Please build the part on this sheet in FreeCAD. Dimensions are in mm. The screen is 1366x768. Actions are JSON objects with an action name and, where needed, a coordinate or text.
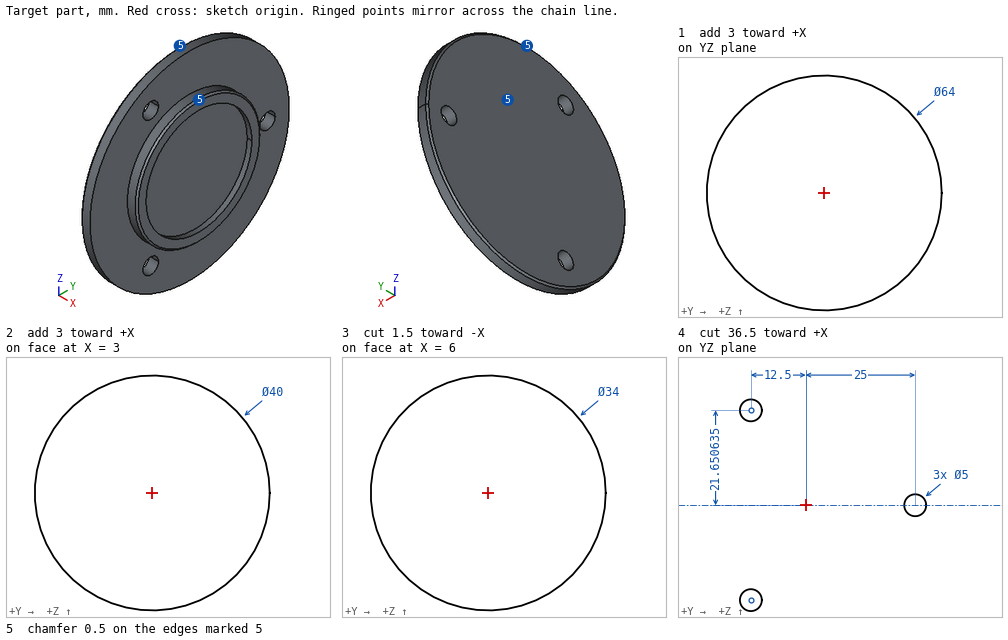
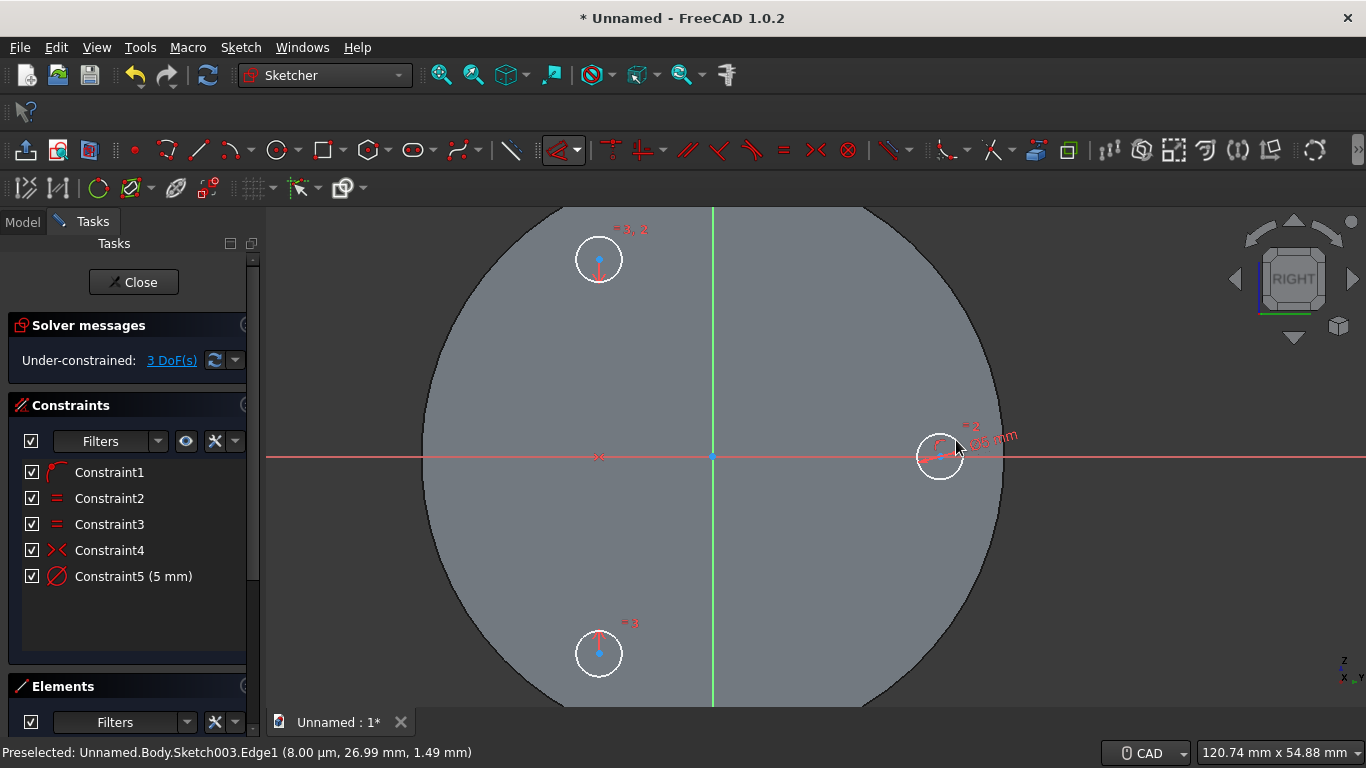
{"action": "left_click", "coordinate": [940, 457]}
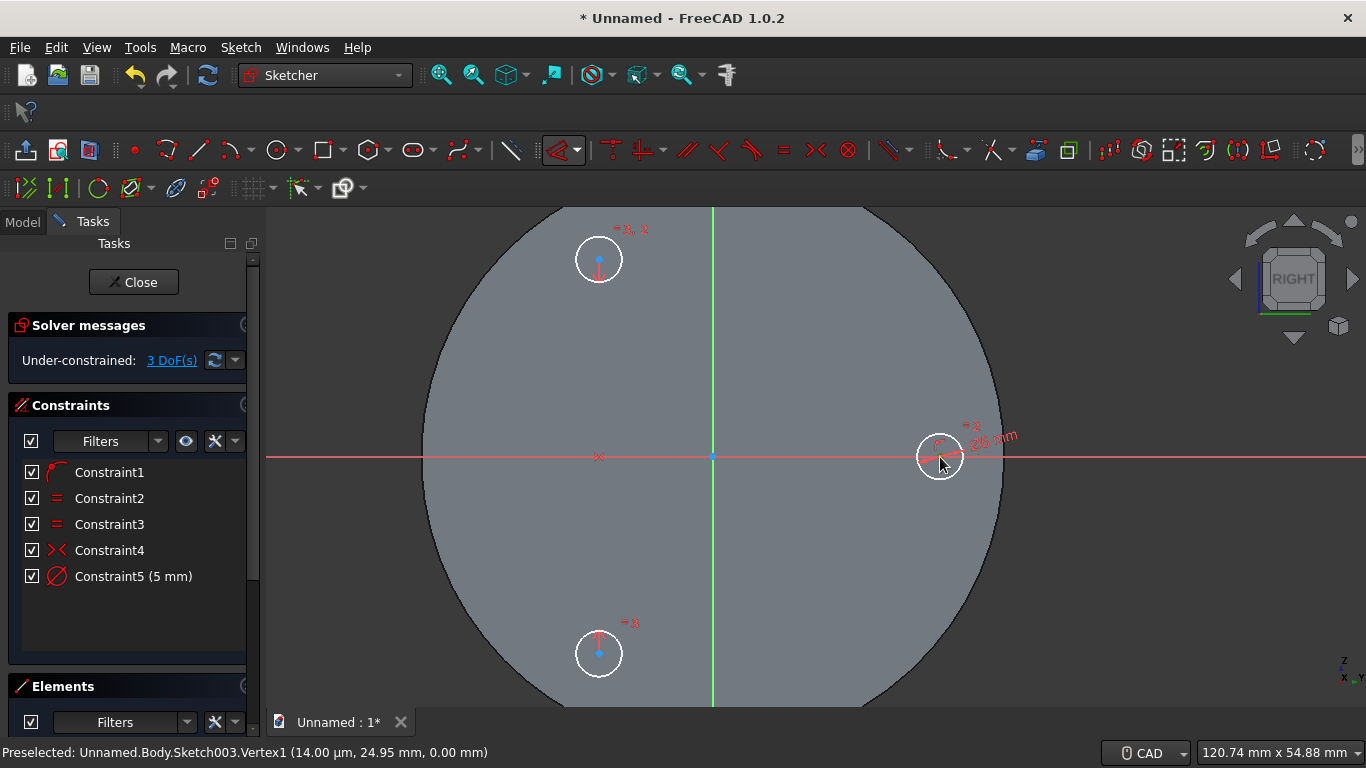
{"action": "key", "text": "l"}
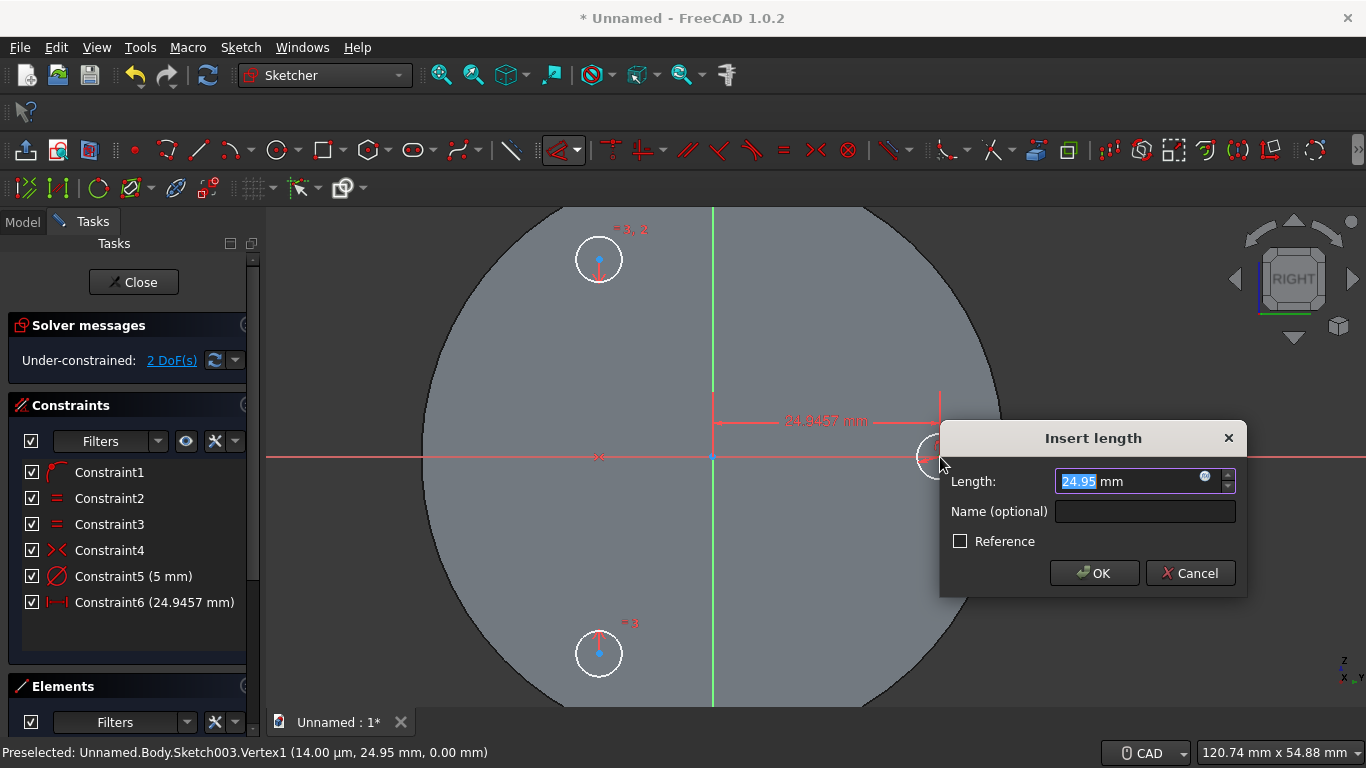
{"action": "type", "text": "25"}
{"action": "key", "text": "Return"}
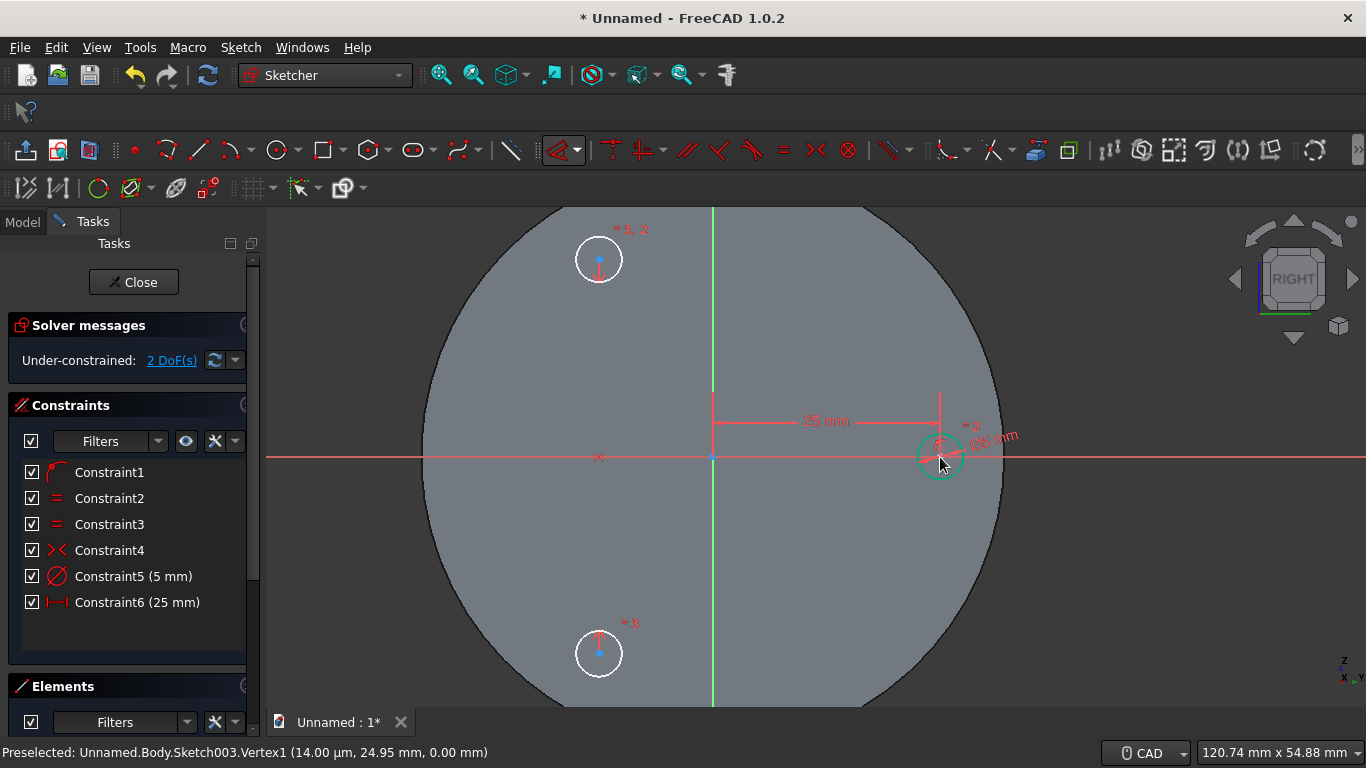
{"action": "left_click", "coordinate": [599, 259]}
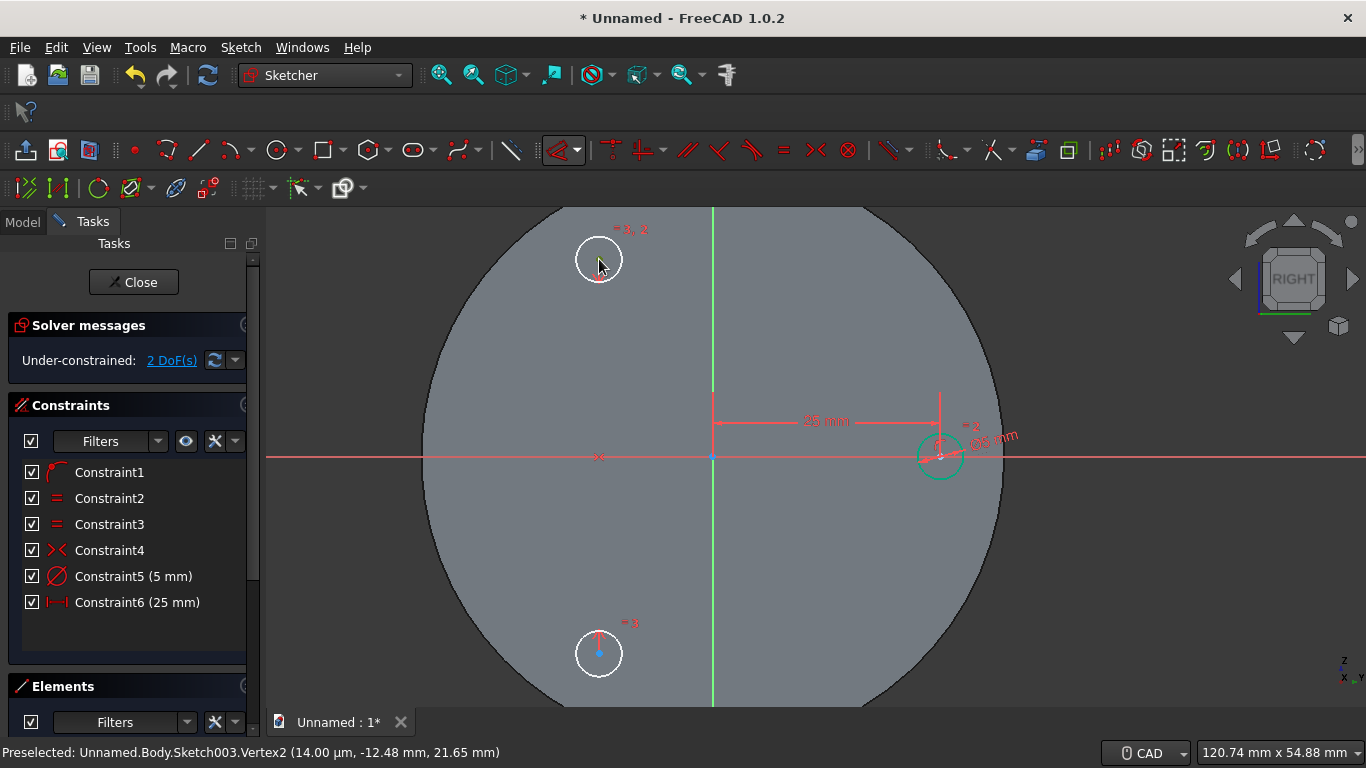
{"action": "left_click", "coordinate": [580, 150]}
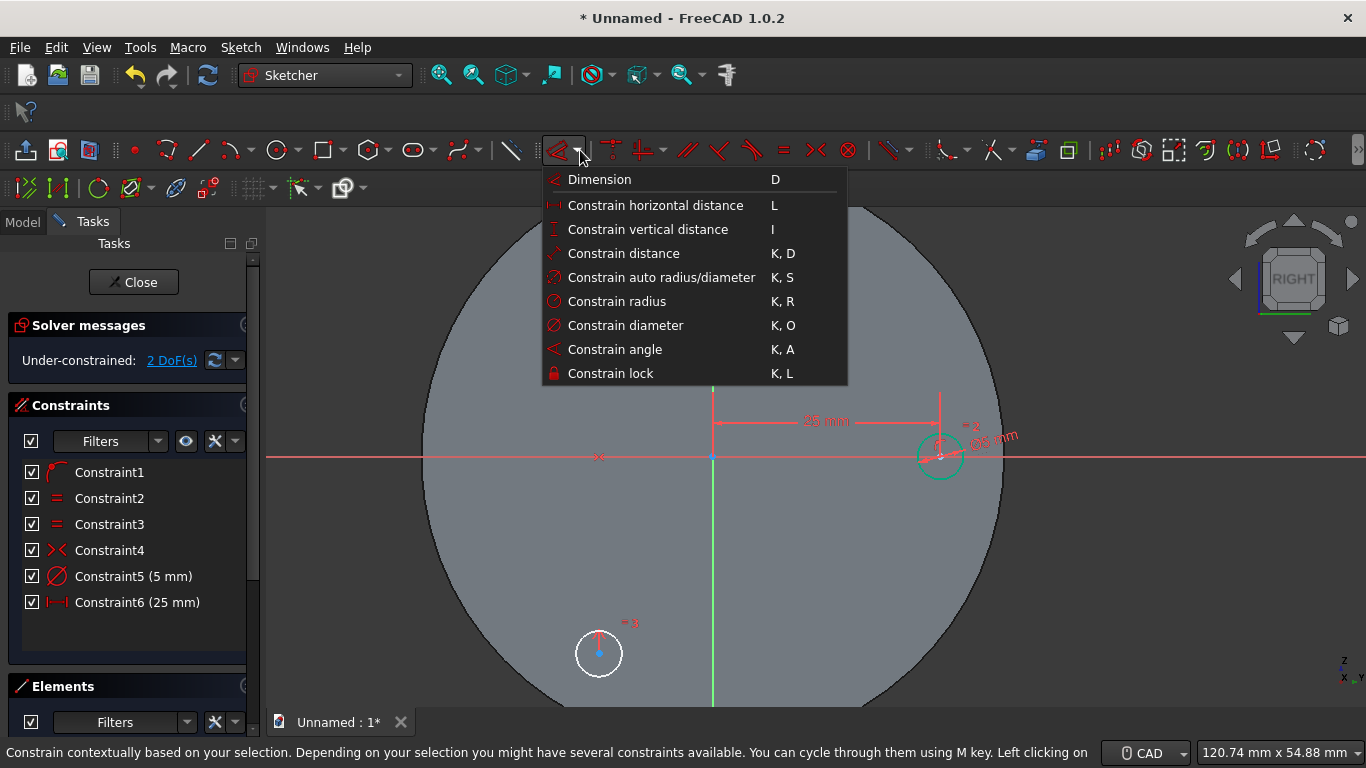
{"action": "left_click", "coordinate": [695, 205]}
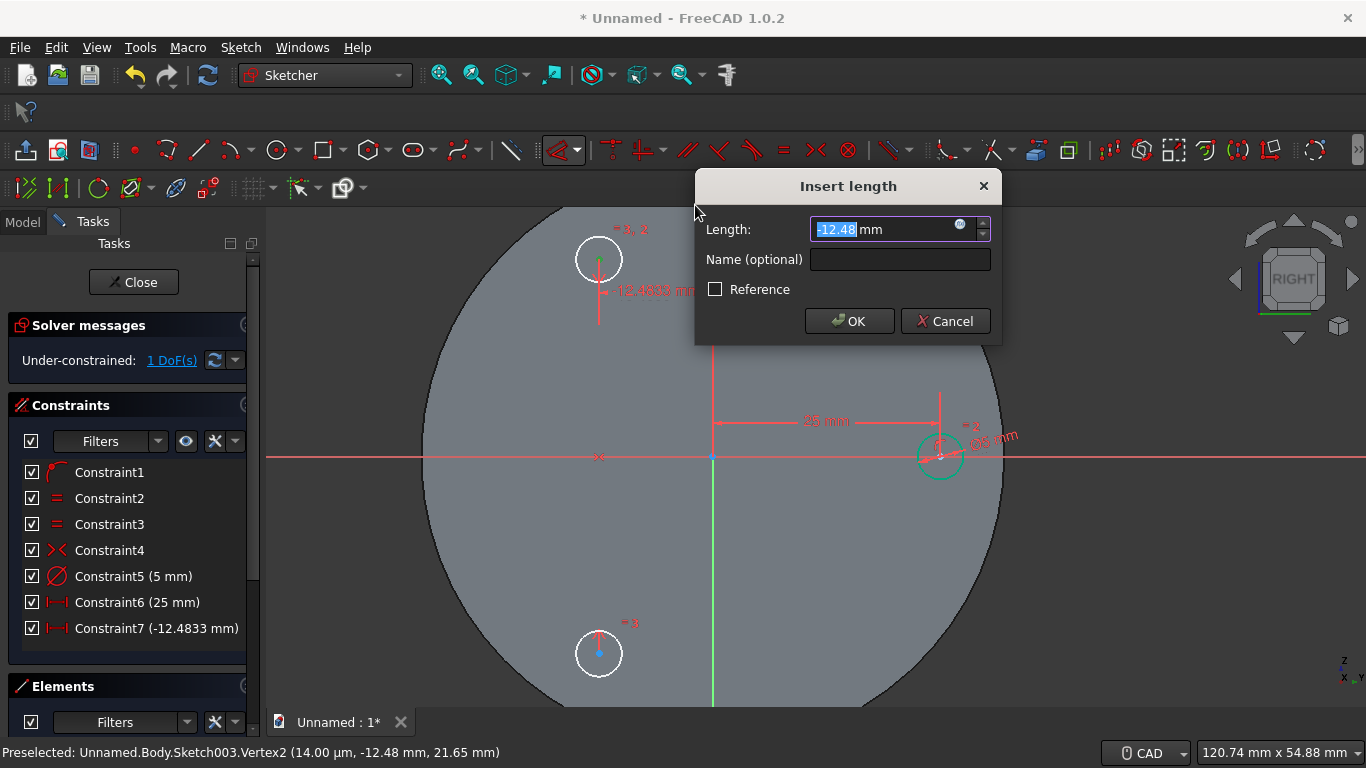
{"action": "type", "text": "-12.5"}
{"action": "key", "text": "Return"}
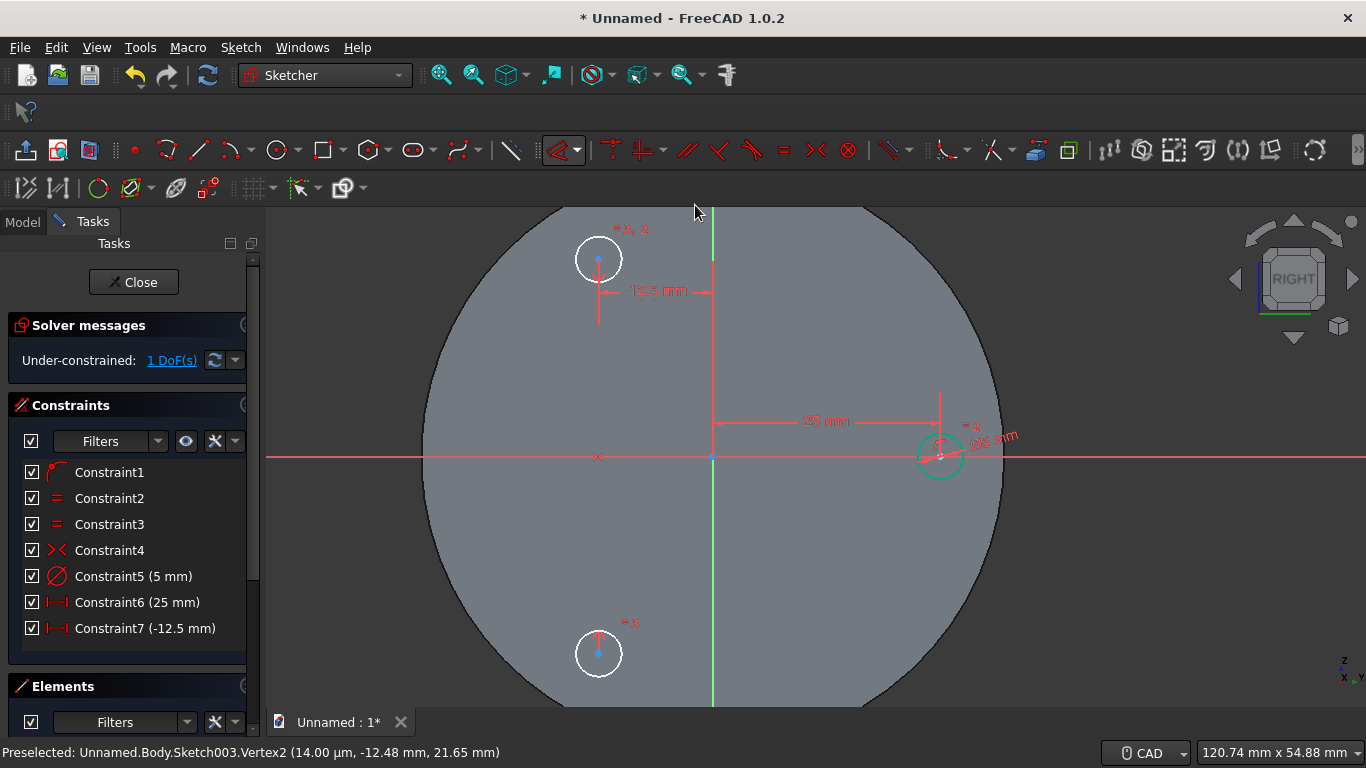
{"action": "left_click", "coordinate": [599, 259]}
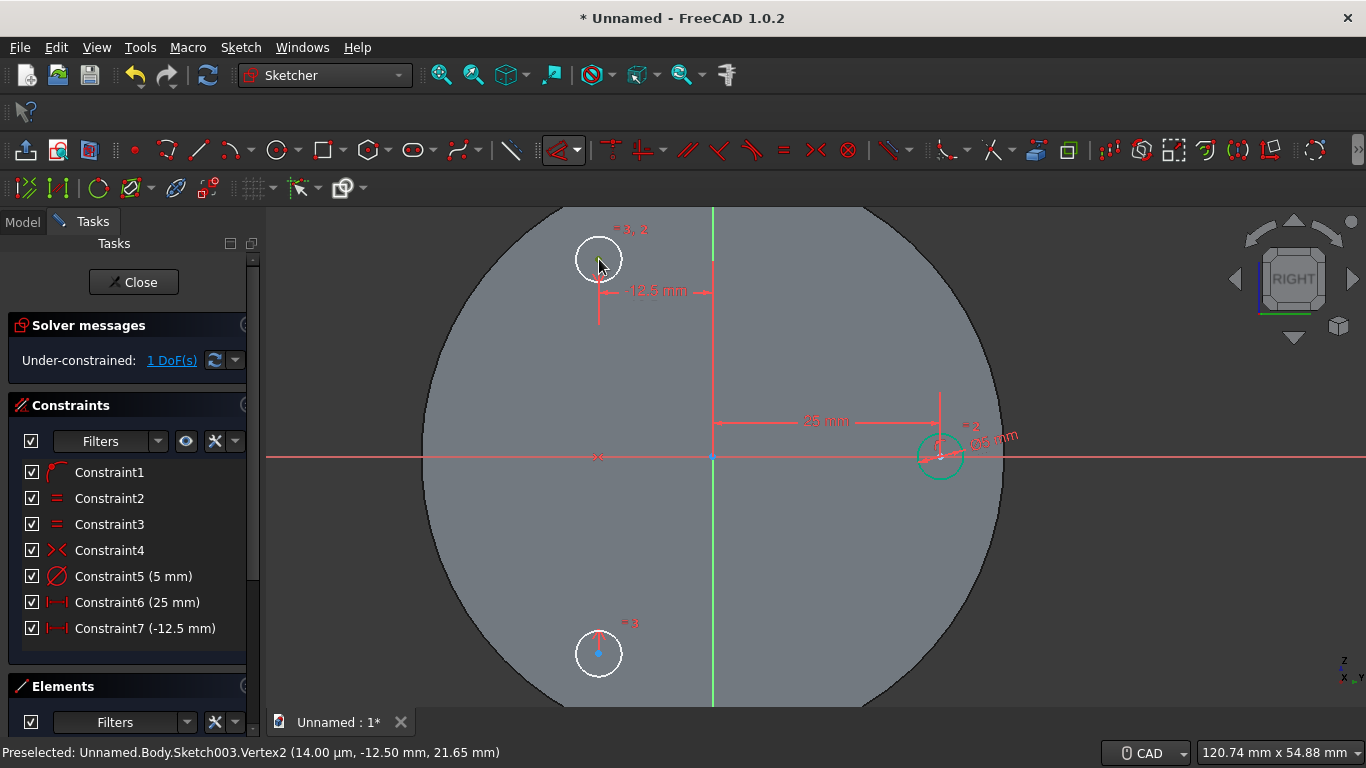
{"action": "key", "text": "i"}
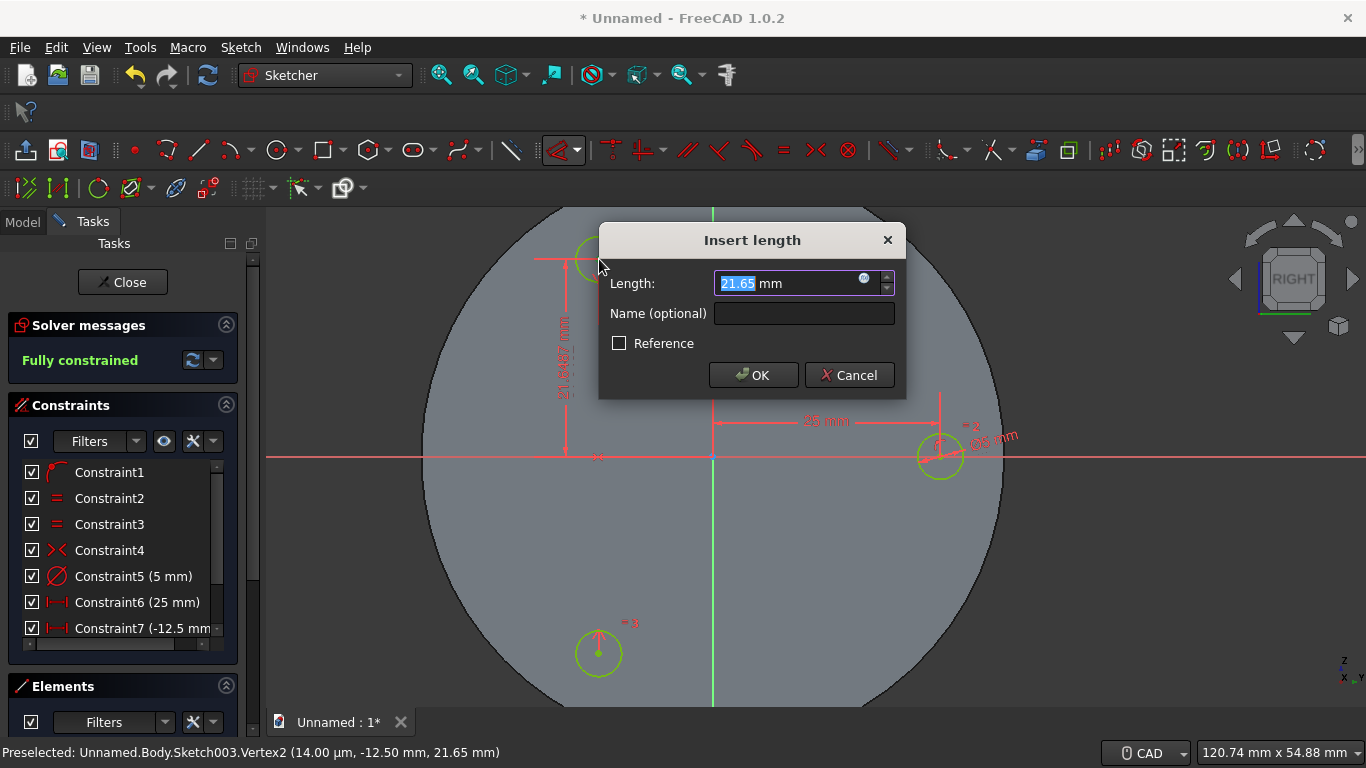
{"action": "type", "text": "21.650635"}
{"action": "key", "text": "Return"}